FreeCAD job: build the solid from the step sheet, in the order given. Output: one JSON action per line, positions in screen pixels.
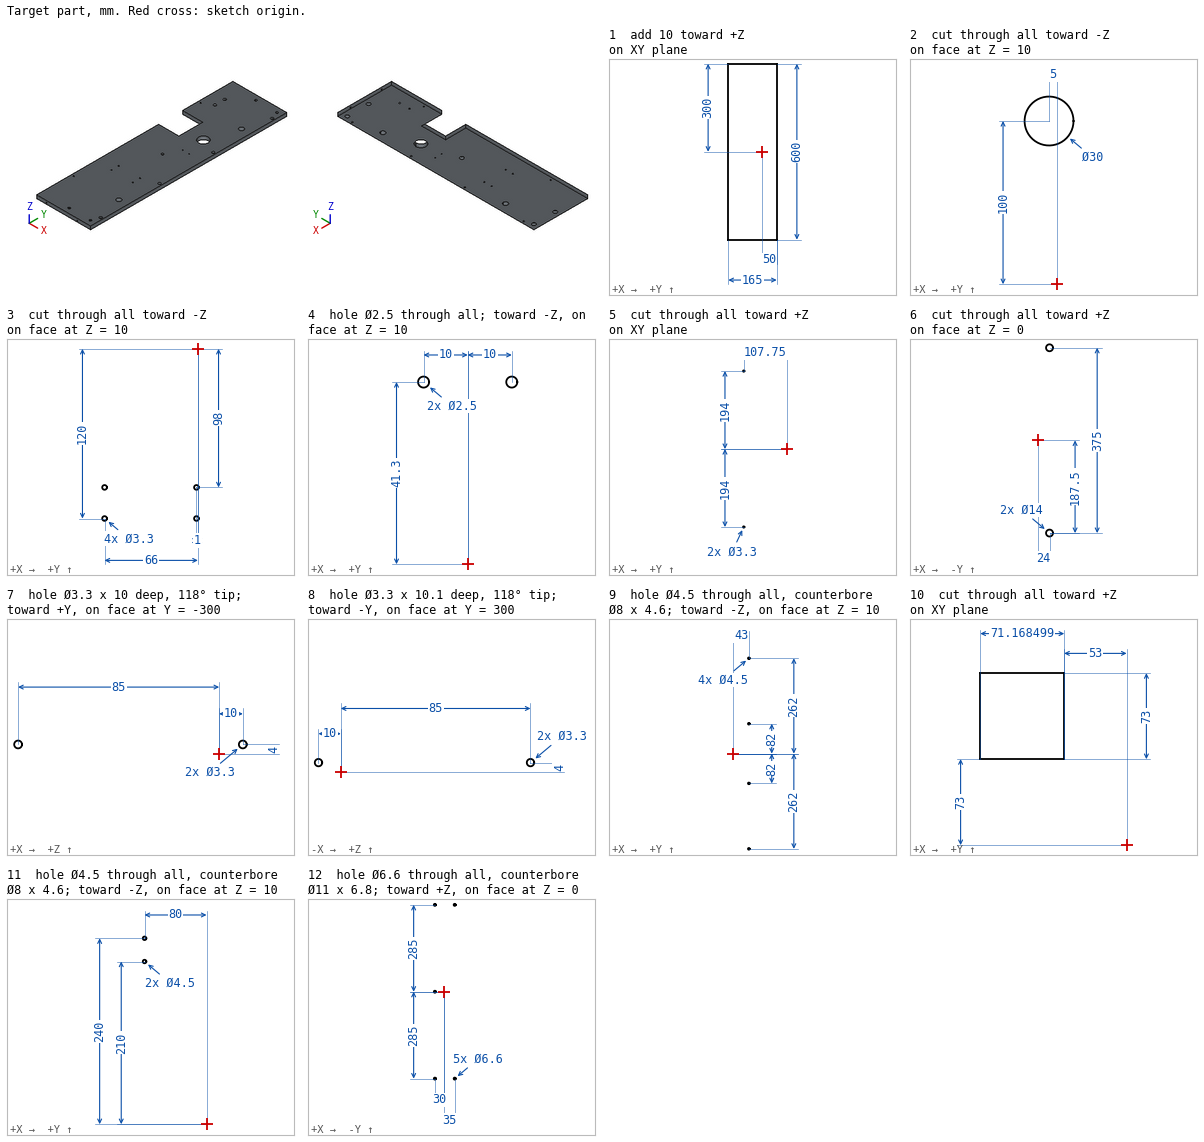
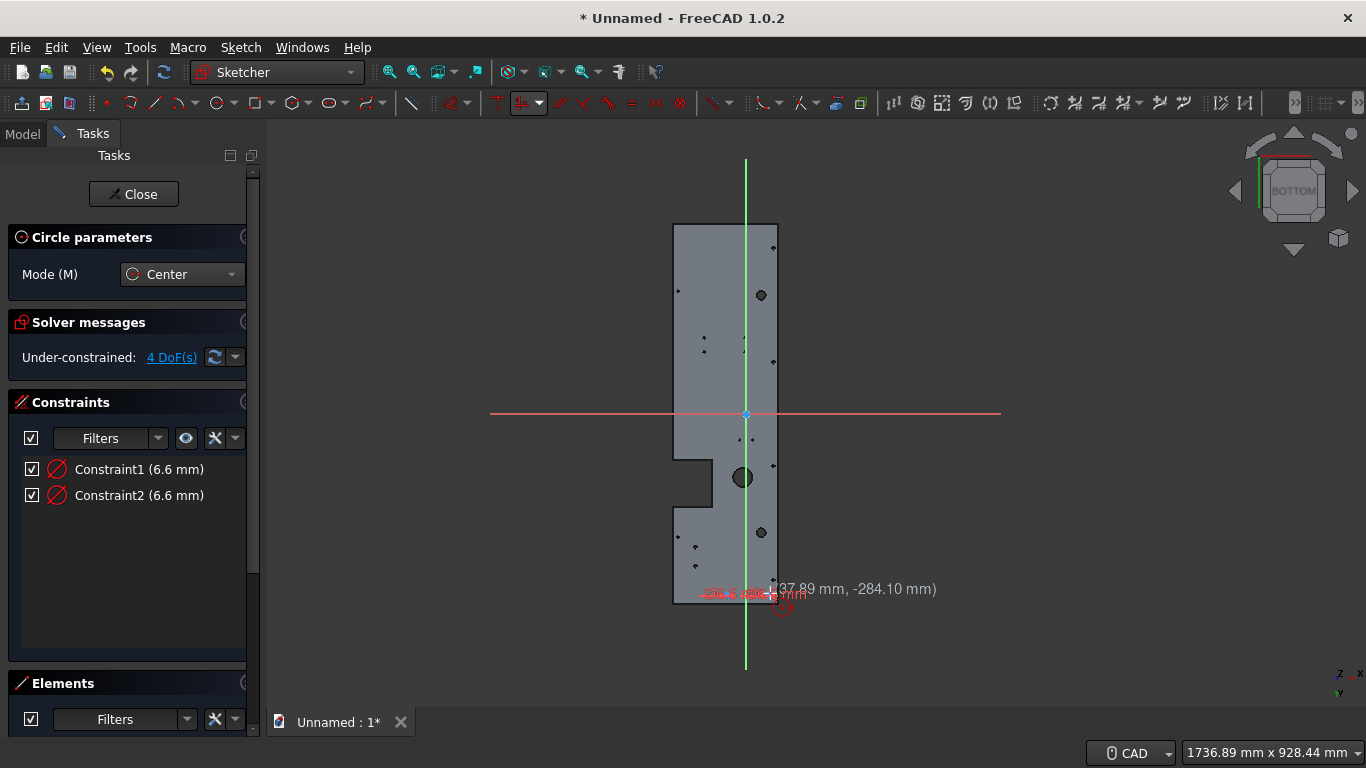
{"action": "scroll", "coordinate": [727, 414], "scroll_direction": "up", "scroll_amount": 12}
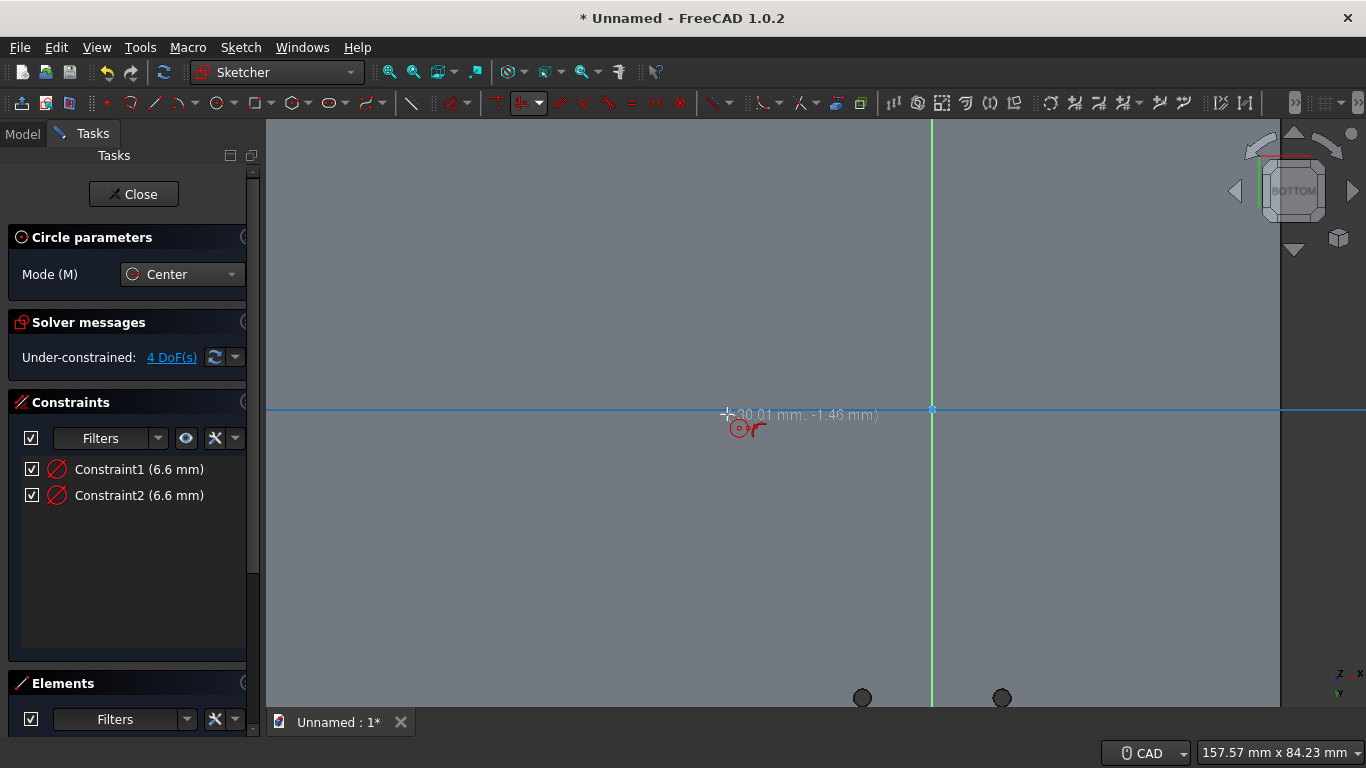
{"action": "scroll", "coordinate": [727, 413], "scroll_direction": "down", "scroll_amount": 12}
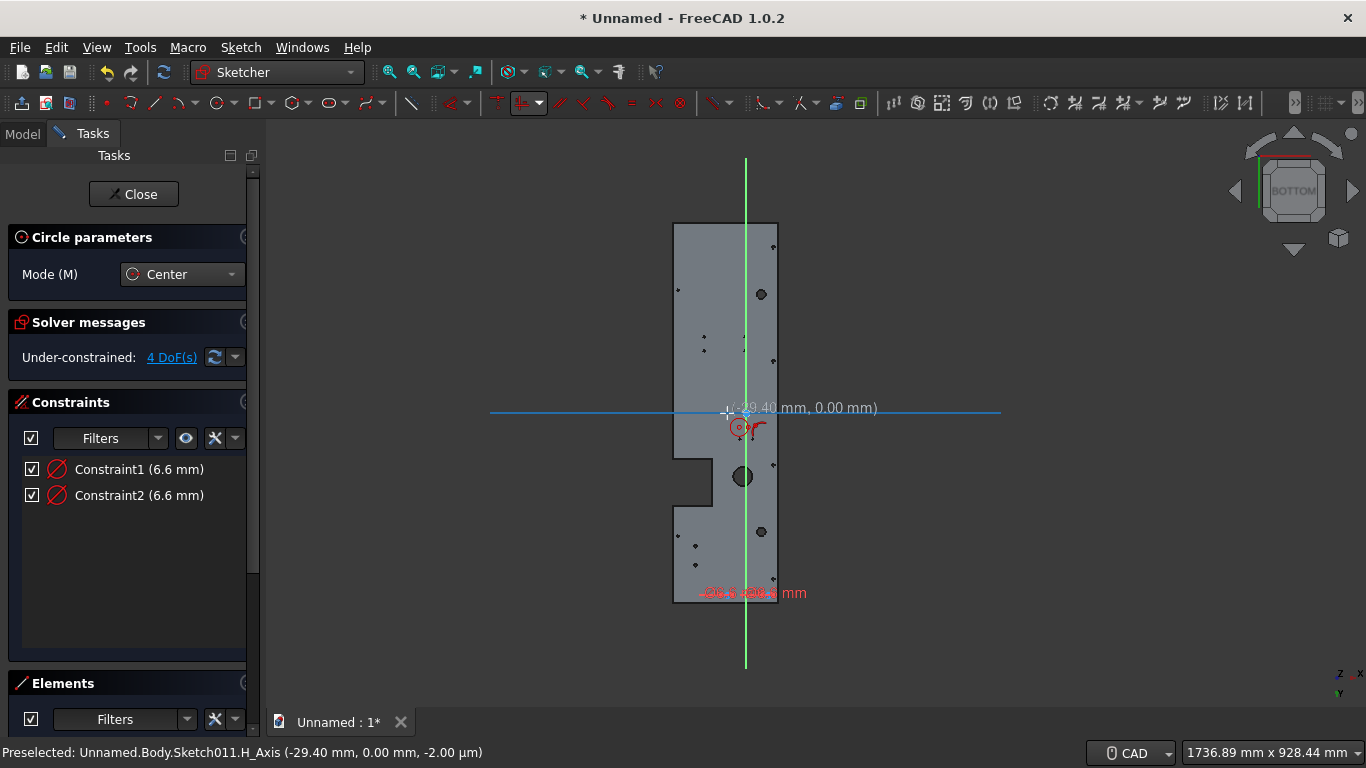
{"action": "left_click", "coordinate": [727, 413]}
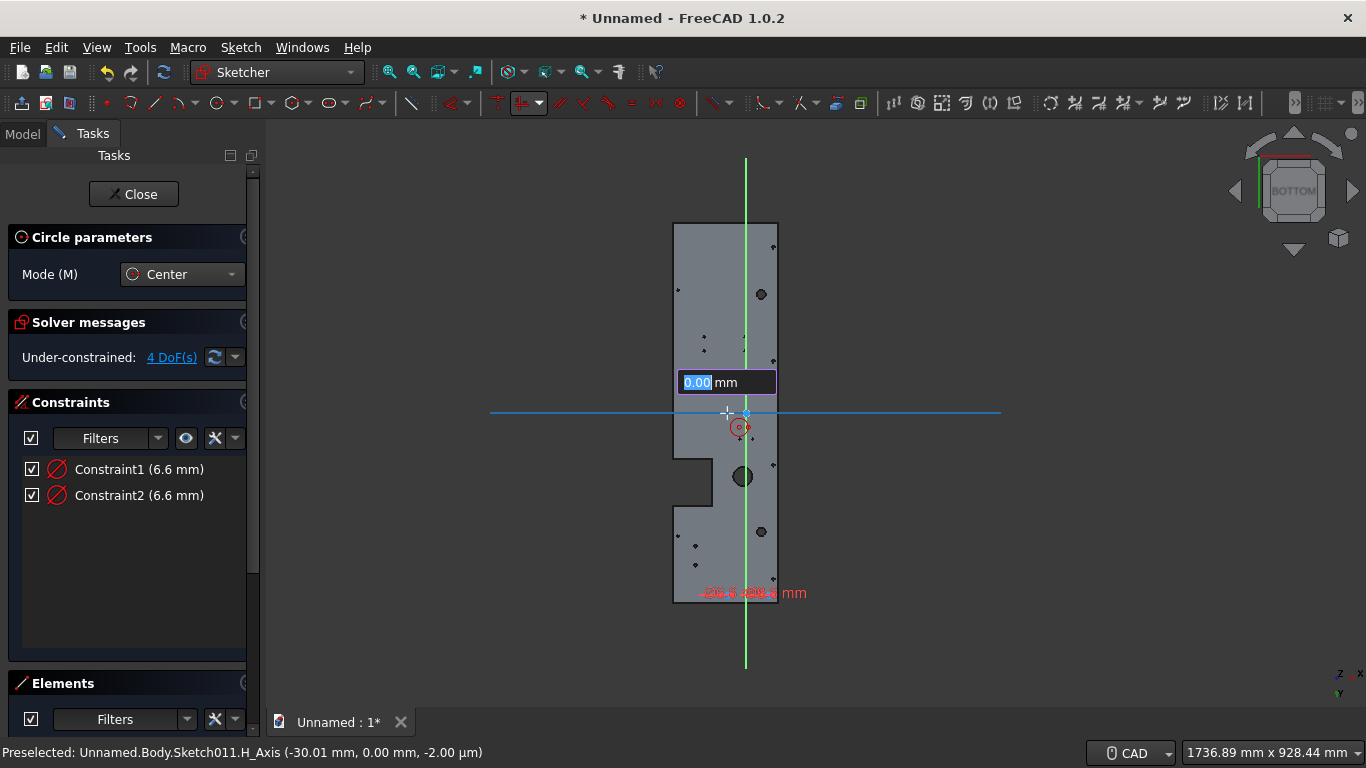
{"action": "scroll", "coordinate": [726, 415], "scroll_direction": "up", "scroll_amount": 11}
{"action": "mouse_move", "coordinate": [725, 412]}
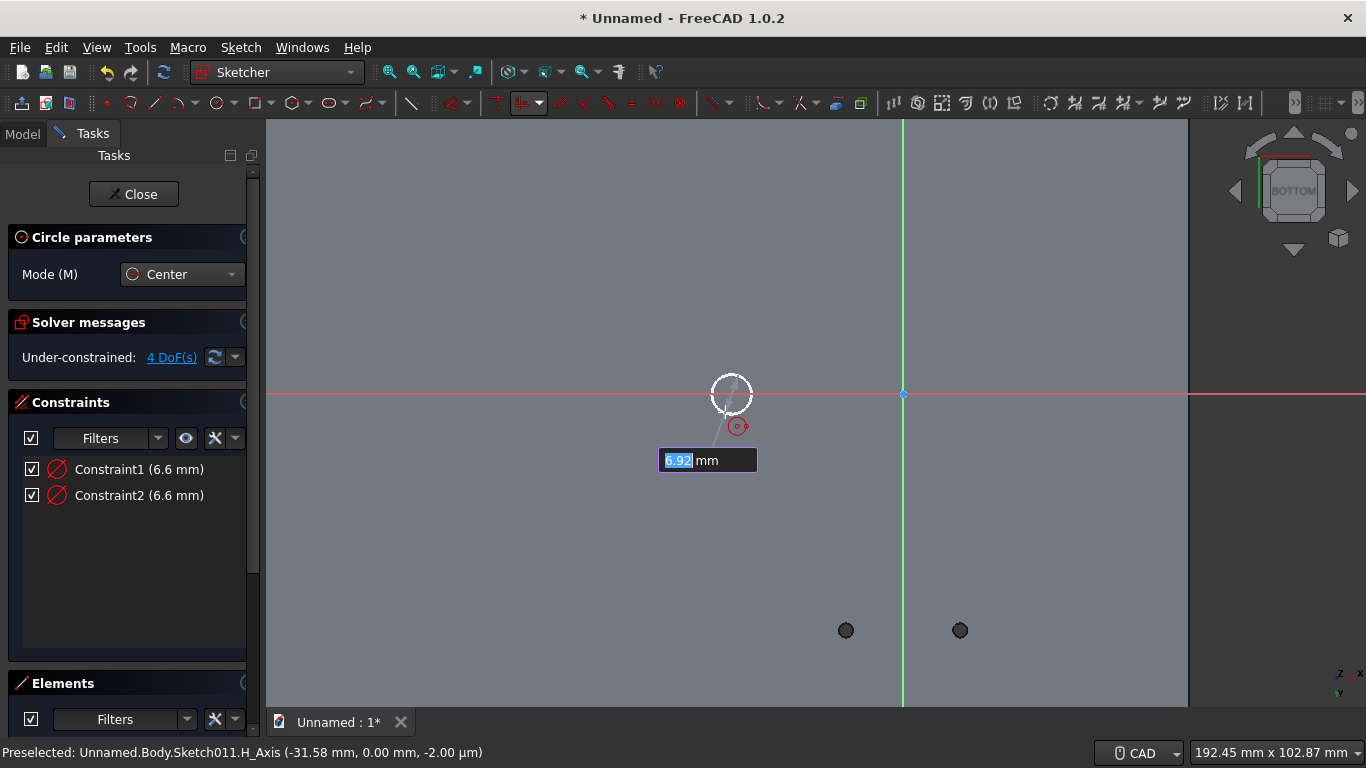
{"action": "type", "text": "6.6"}
{"action": "key", "text": "Return"}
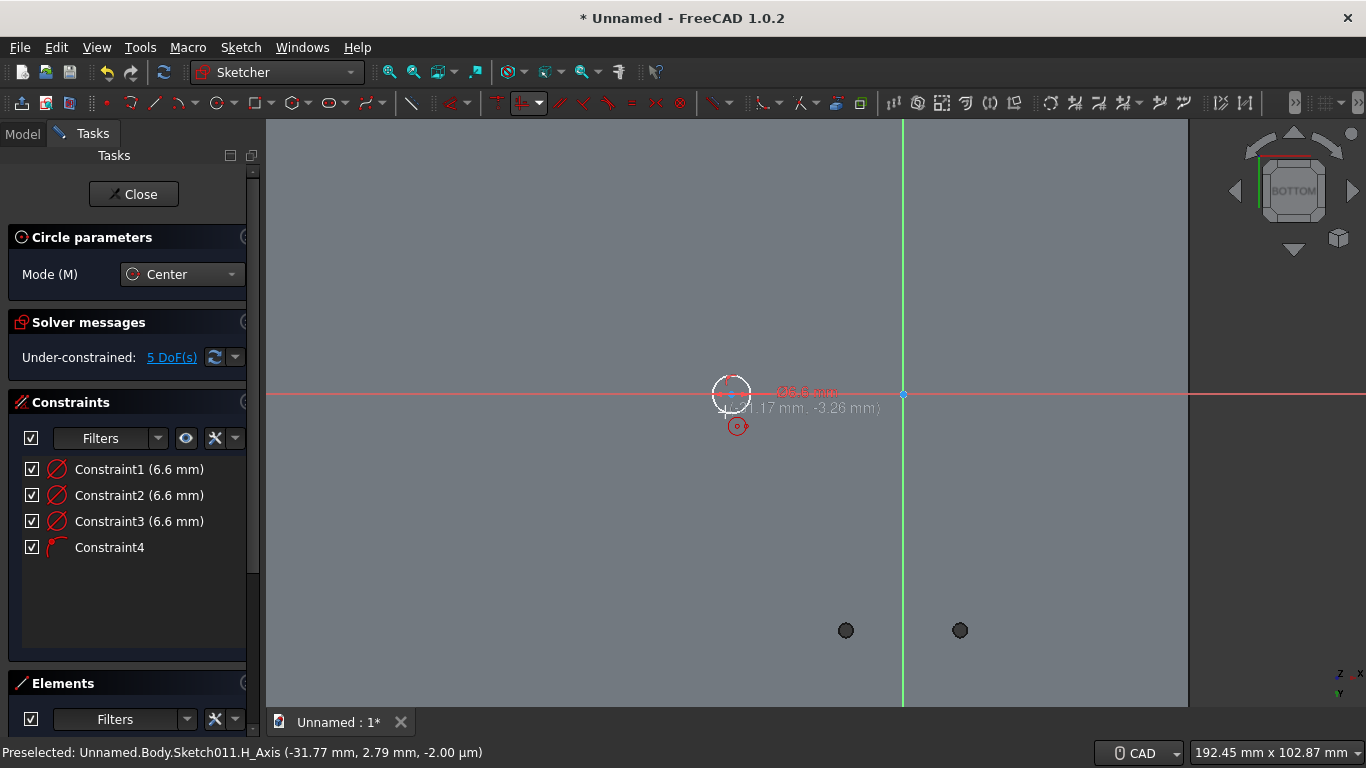
{"action": "scroll", "coordinate": [726, 415], "scroll_direction": "down", "scroll_amount": 11}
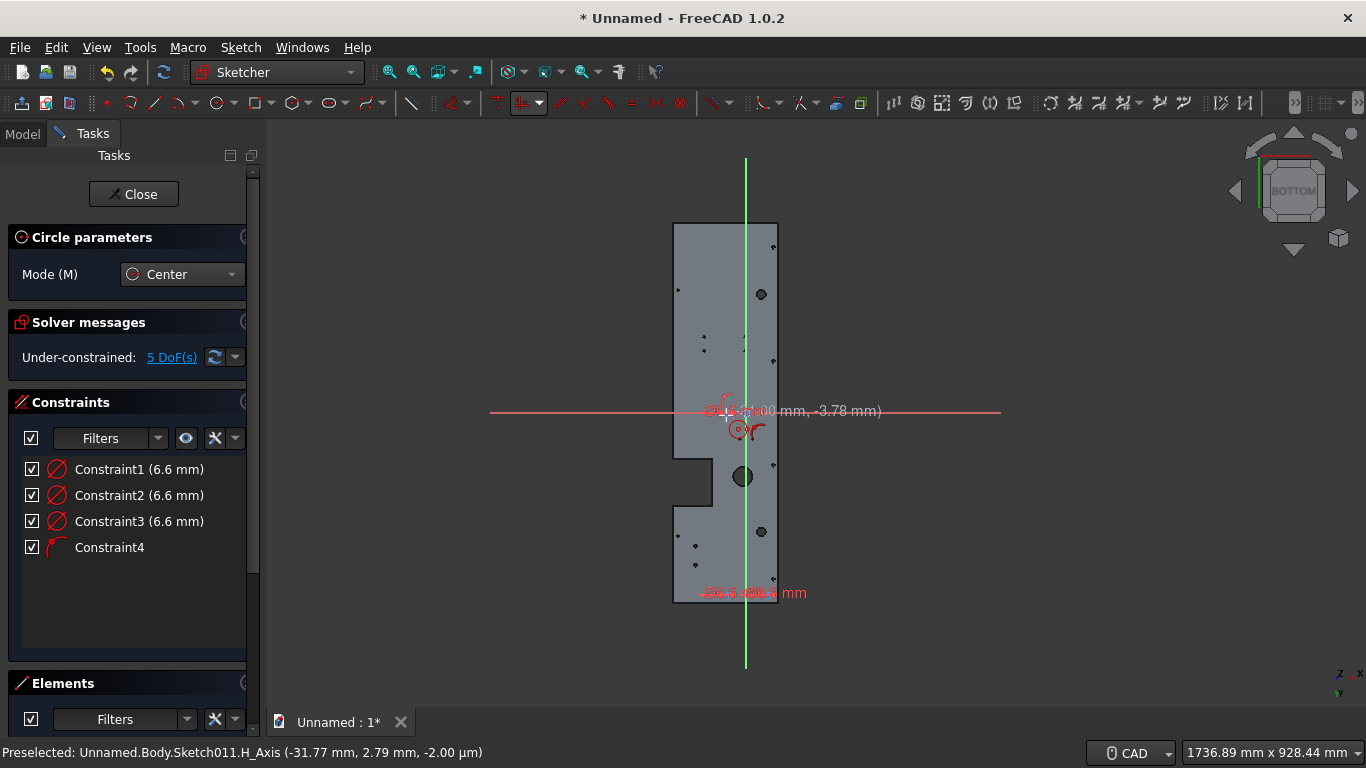
{"action": "scroll", "coordinate": [727, 233], "scroll_direction": "up", "scroll_amount": 12}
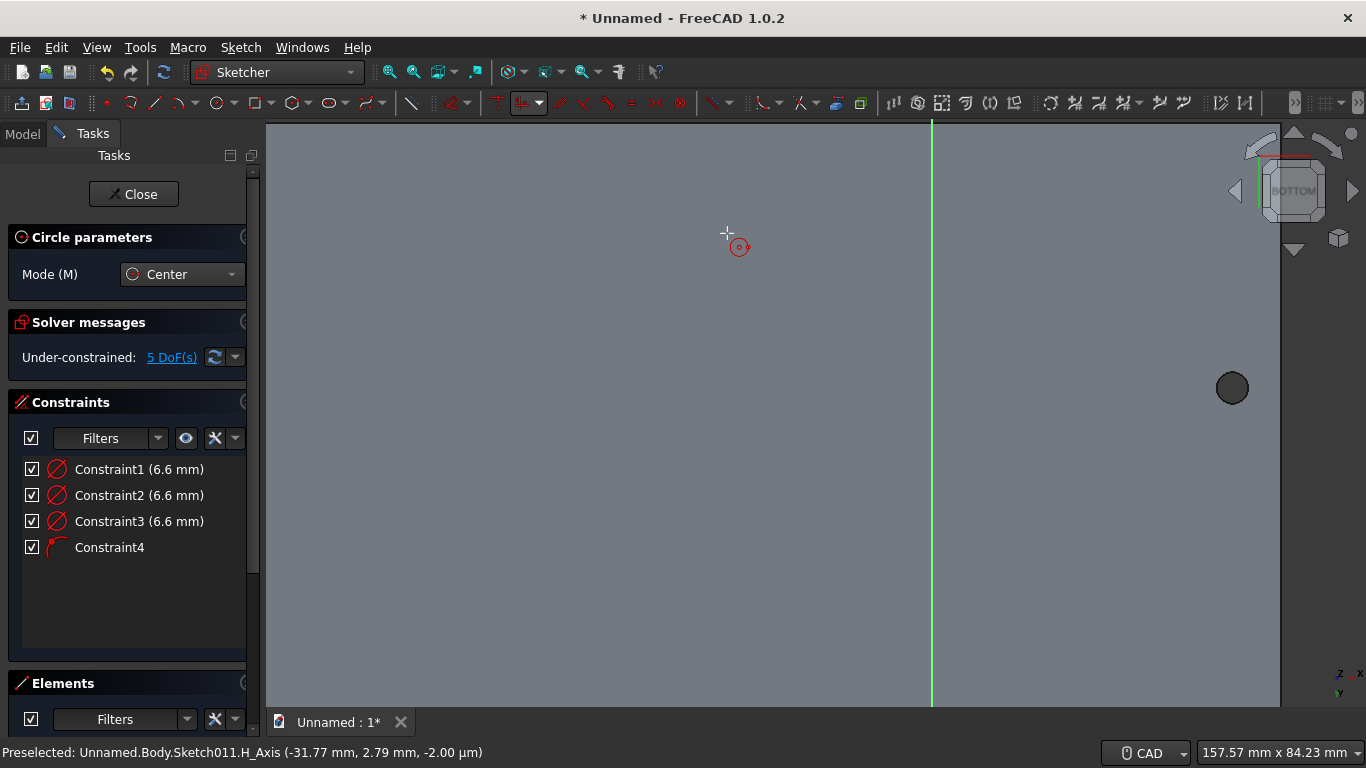
{"action": "scroll", "coordinate": [727, 233], "scroll_direction": "down", "scroll_amount": 12}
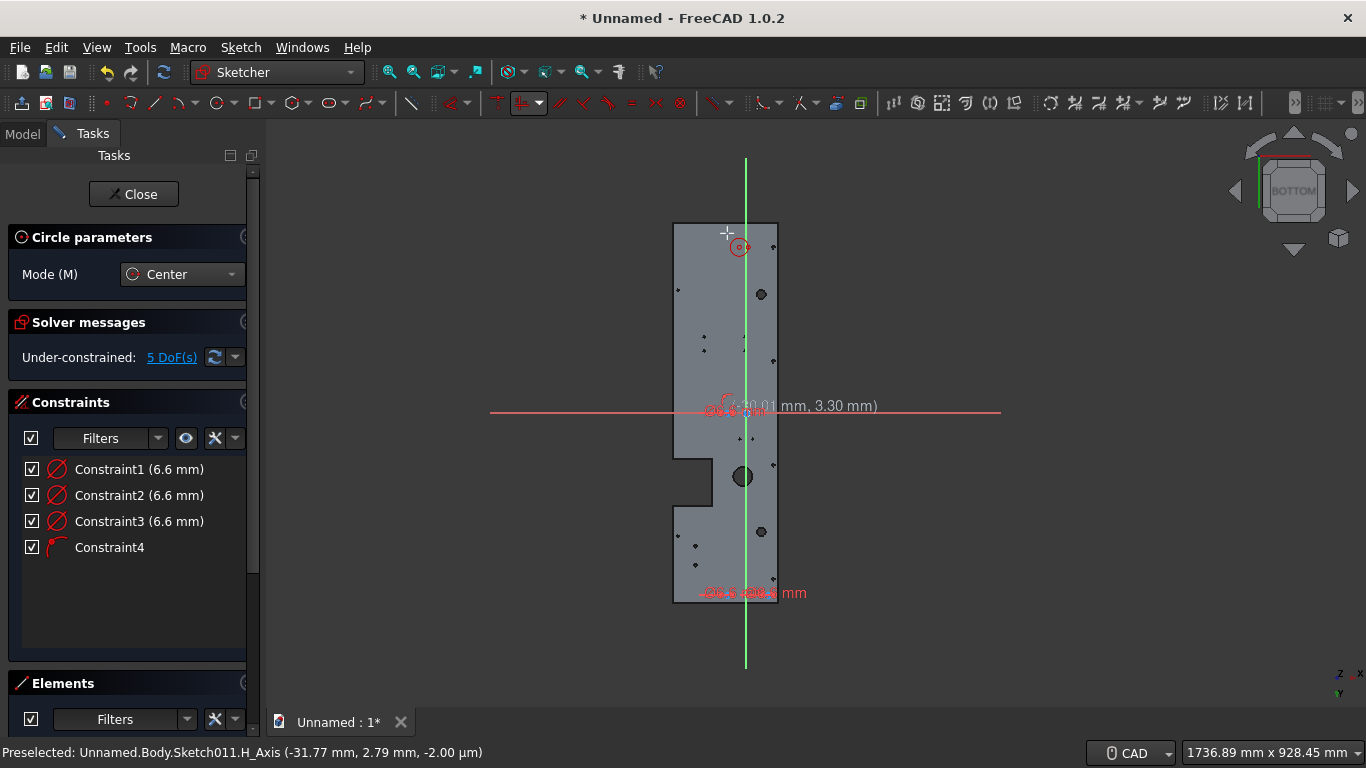
{"action": "left_click", "coordinate": [727, 233]}
{"action": "mouse_move", "coordinate": [728, 231]}